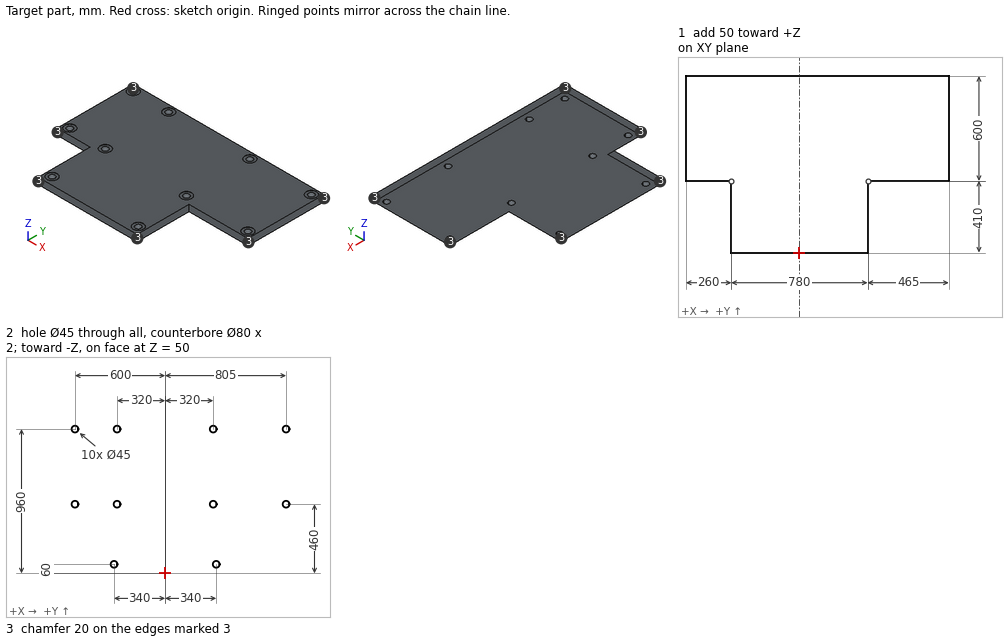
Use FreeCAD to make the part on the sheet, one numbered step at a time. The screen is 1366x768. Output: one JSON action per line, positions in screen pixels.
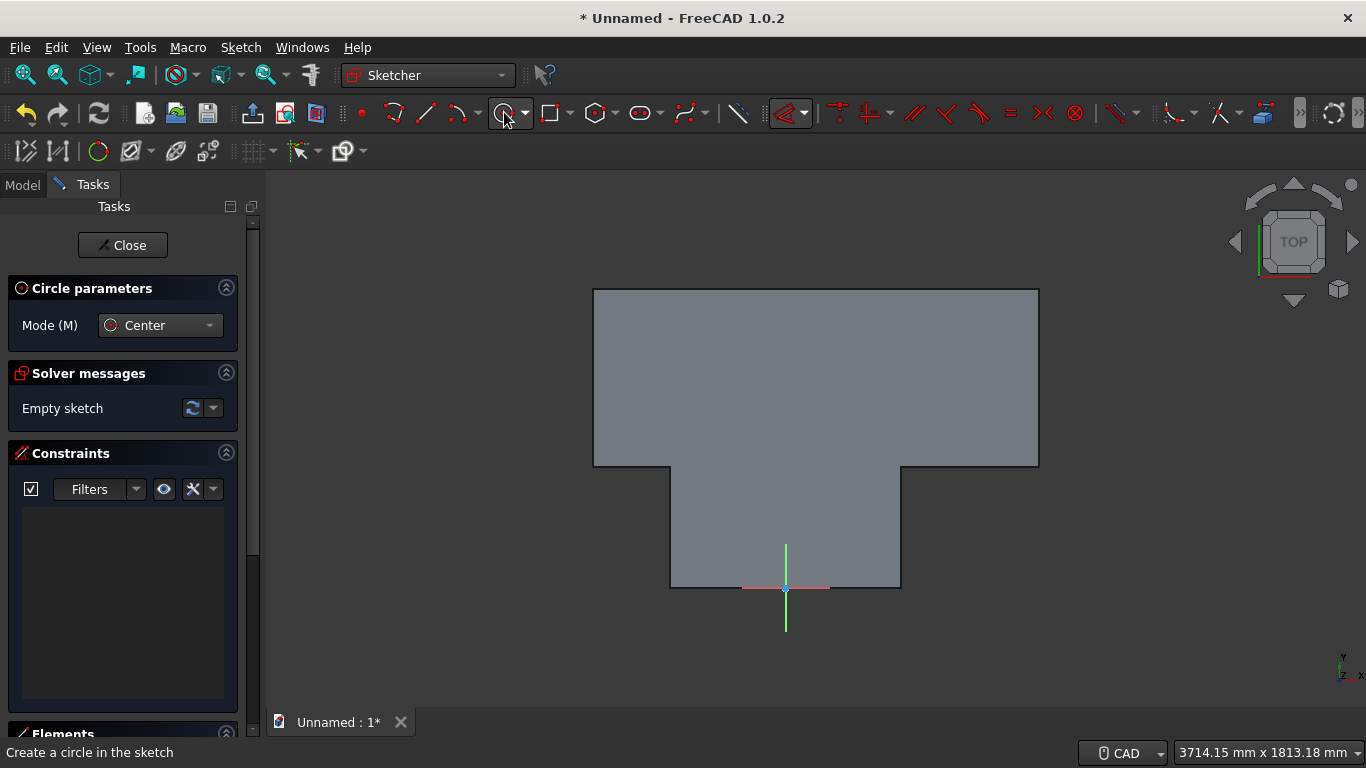
{"action": "scroll", "coordinate": [608, 304], "scroll_direction": "up", "scroll_amount": 7}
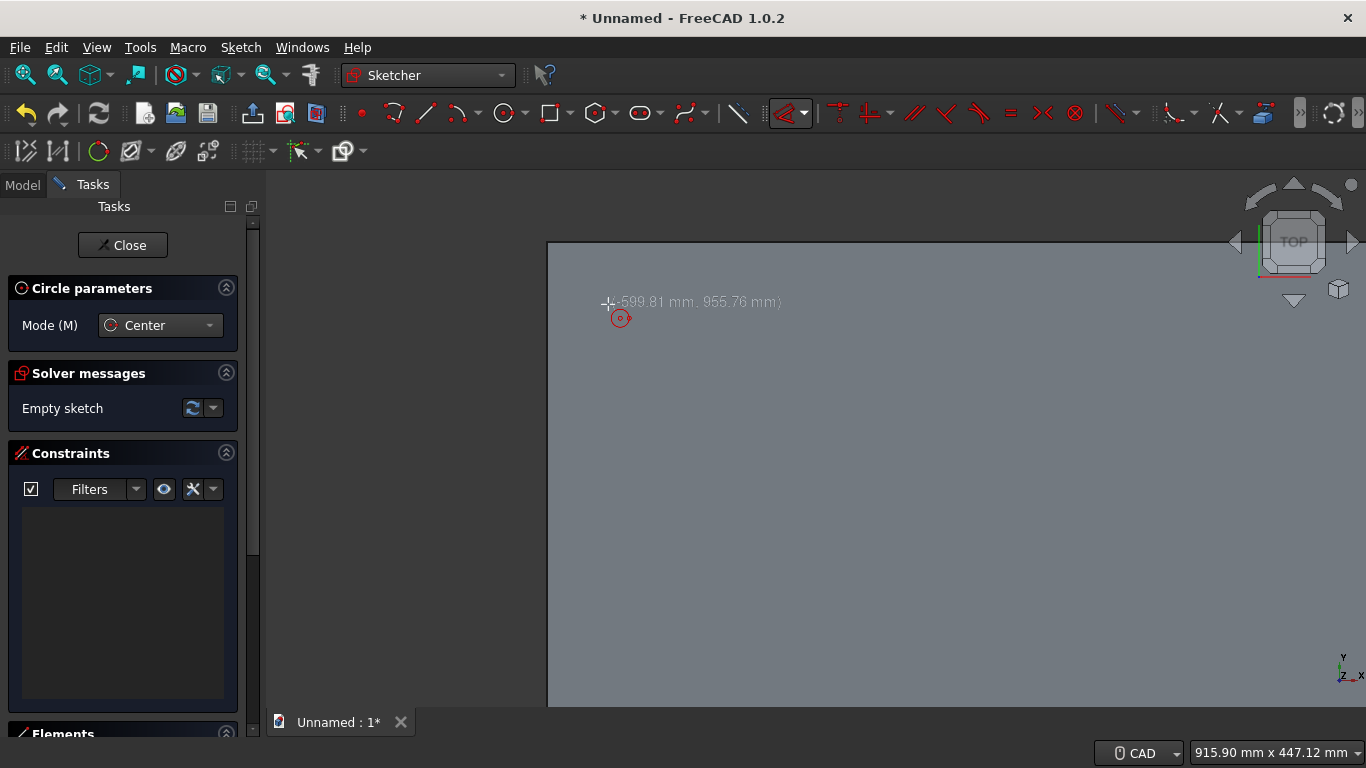
{"action": "scroll", "coordinate": [444, 255], "scroll_direction": "down", "scroll_amount": 6}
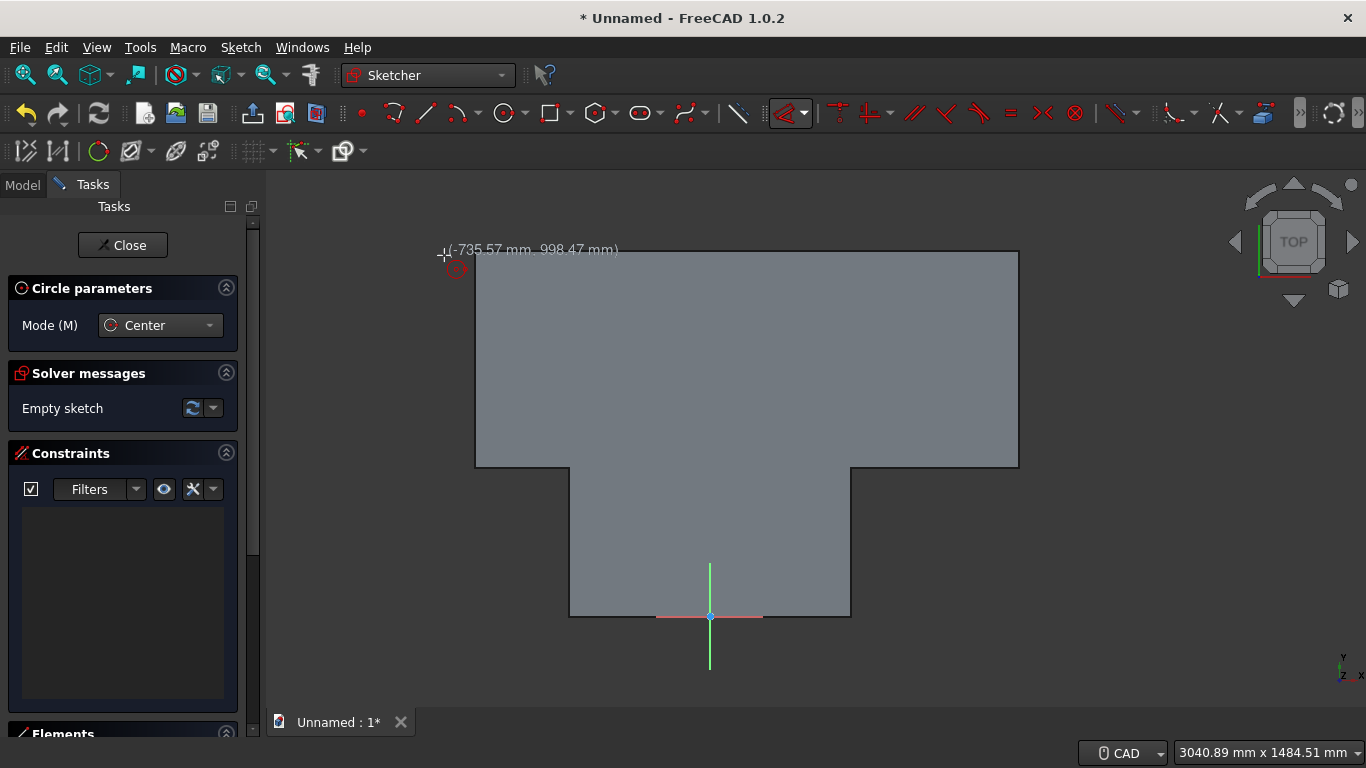
{"action": "left_click", "coordinate": [493, 269]}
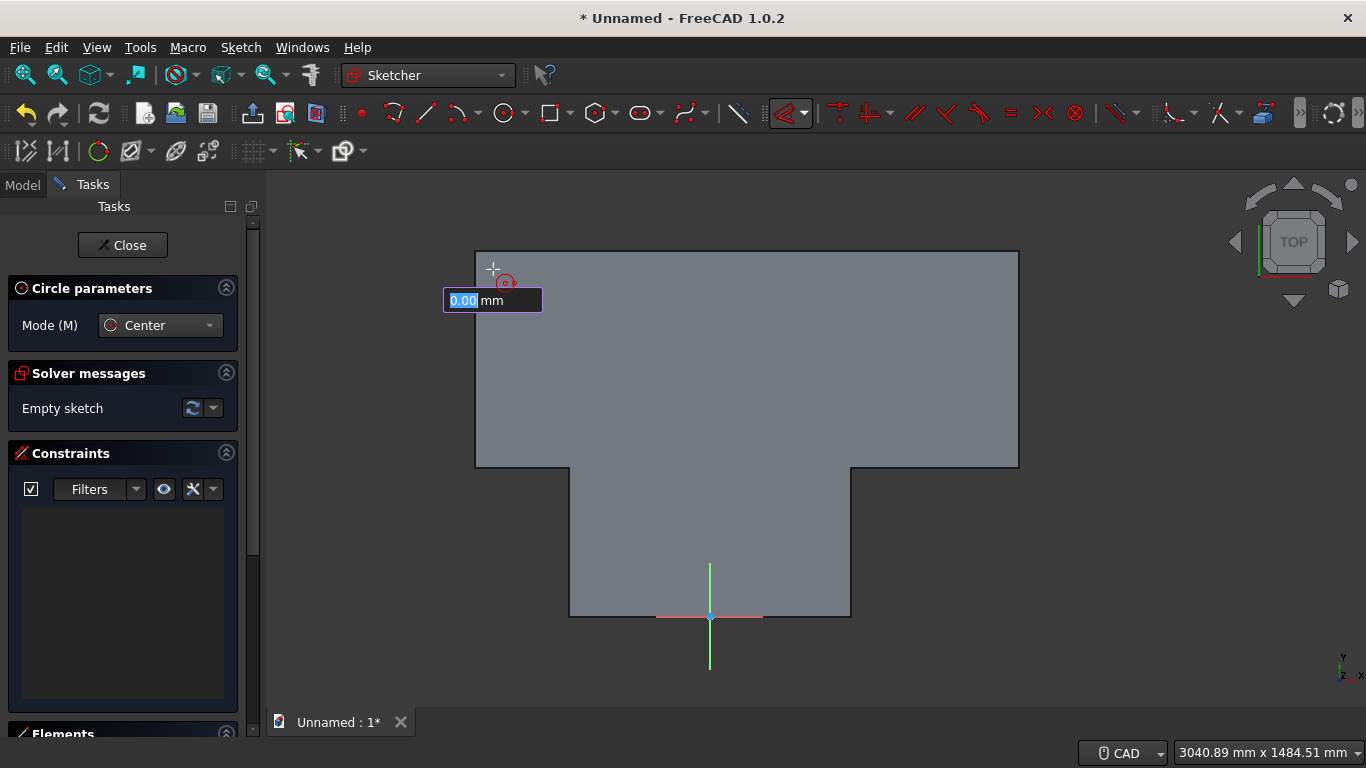
{"action": "scroll", "coordinate": [499, 264], "scroll_direction": "up", "scroll_amount": 4}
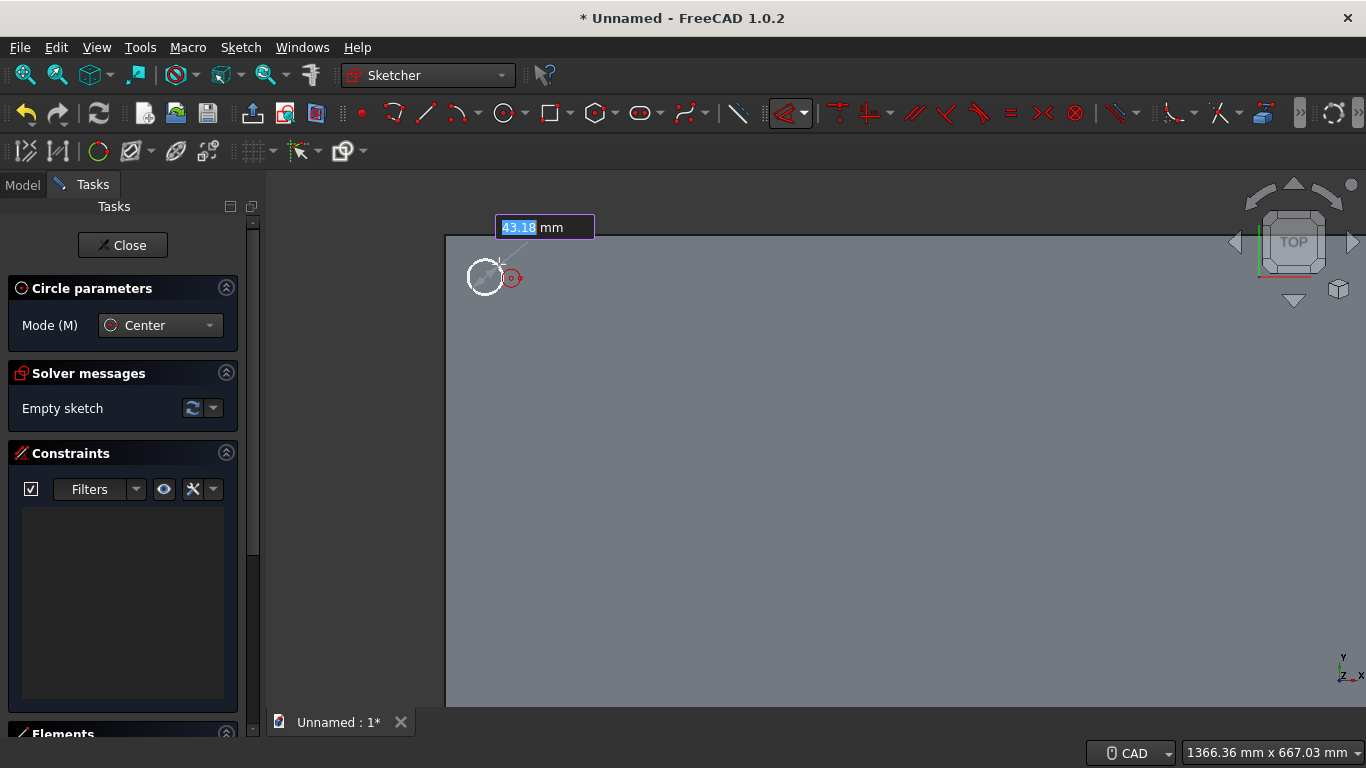
{"action": "left_click", "coordinate": [499, 263]}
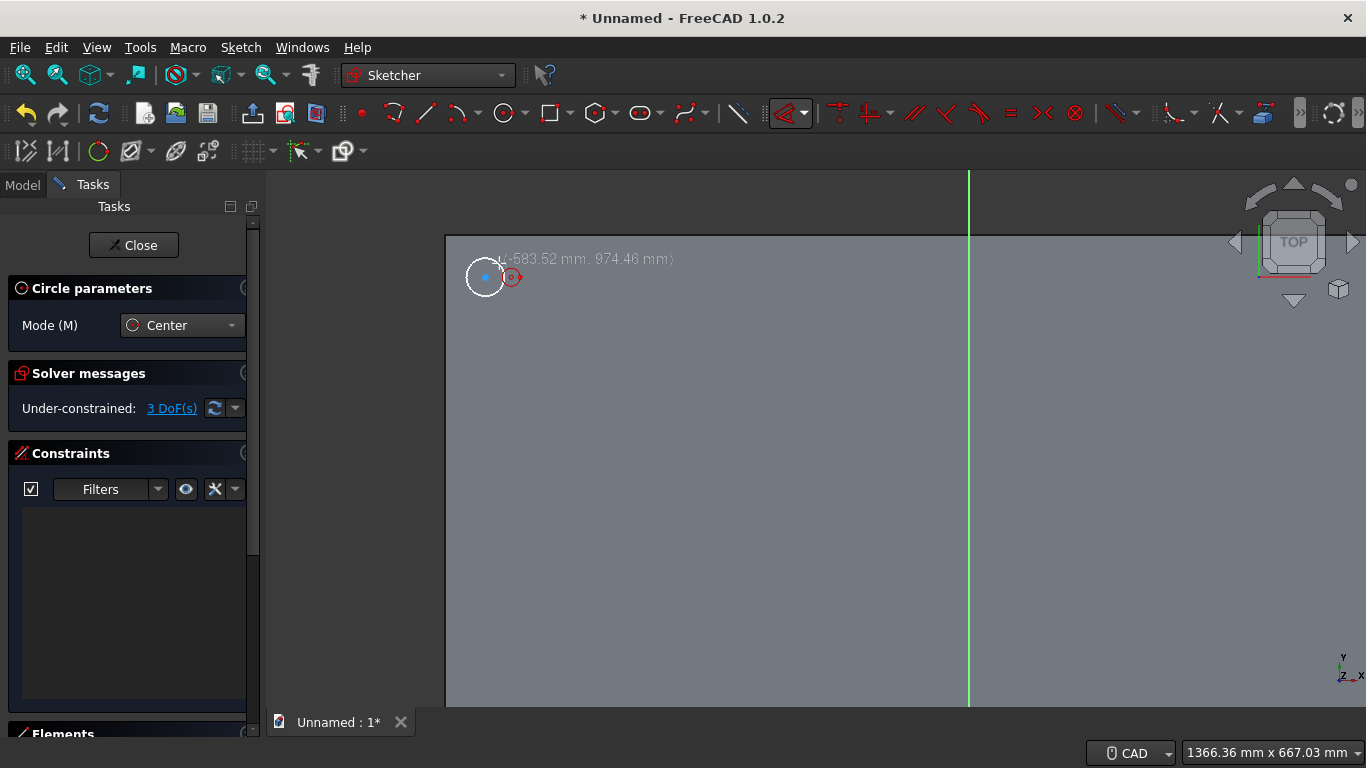
{"action": "scroll", "coordinate": [500, 263], "scroll_direction": "down", "scroll_amount": 4}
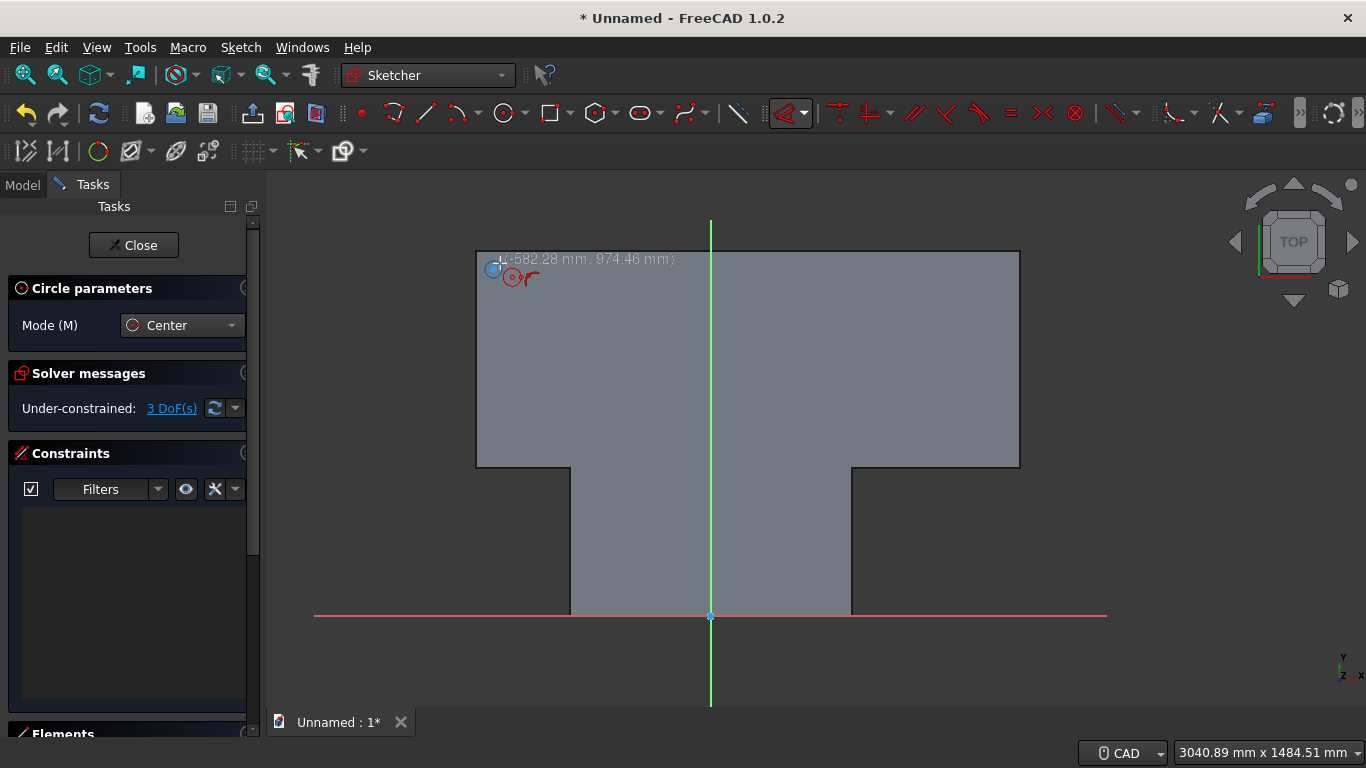
{"action": "scroll", "coordinate": [827, 269], "scroll_direction": "up", "scroll_amount": 6}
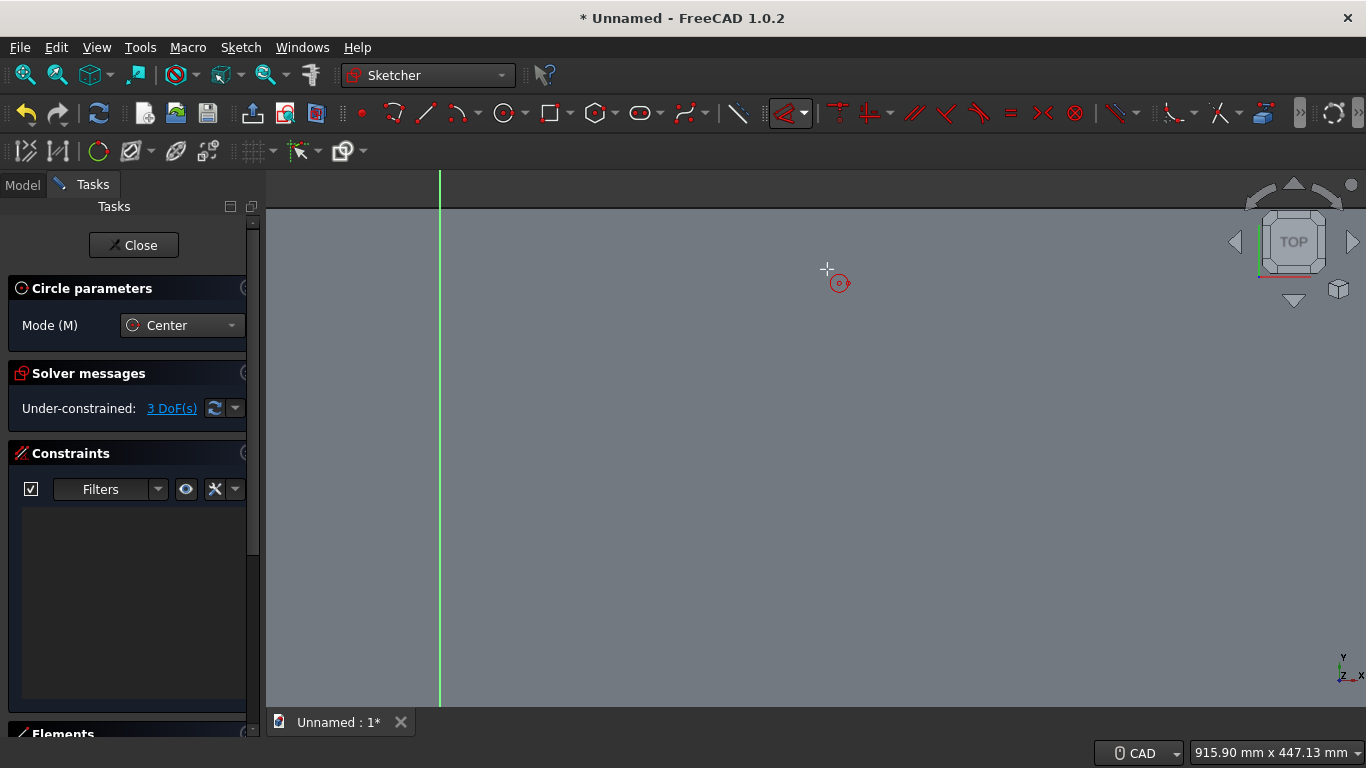
{"action": "scroll", "coordinate": [827, 269], "scroll_direction": "down", "scroll_amount": 6}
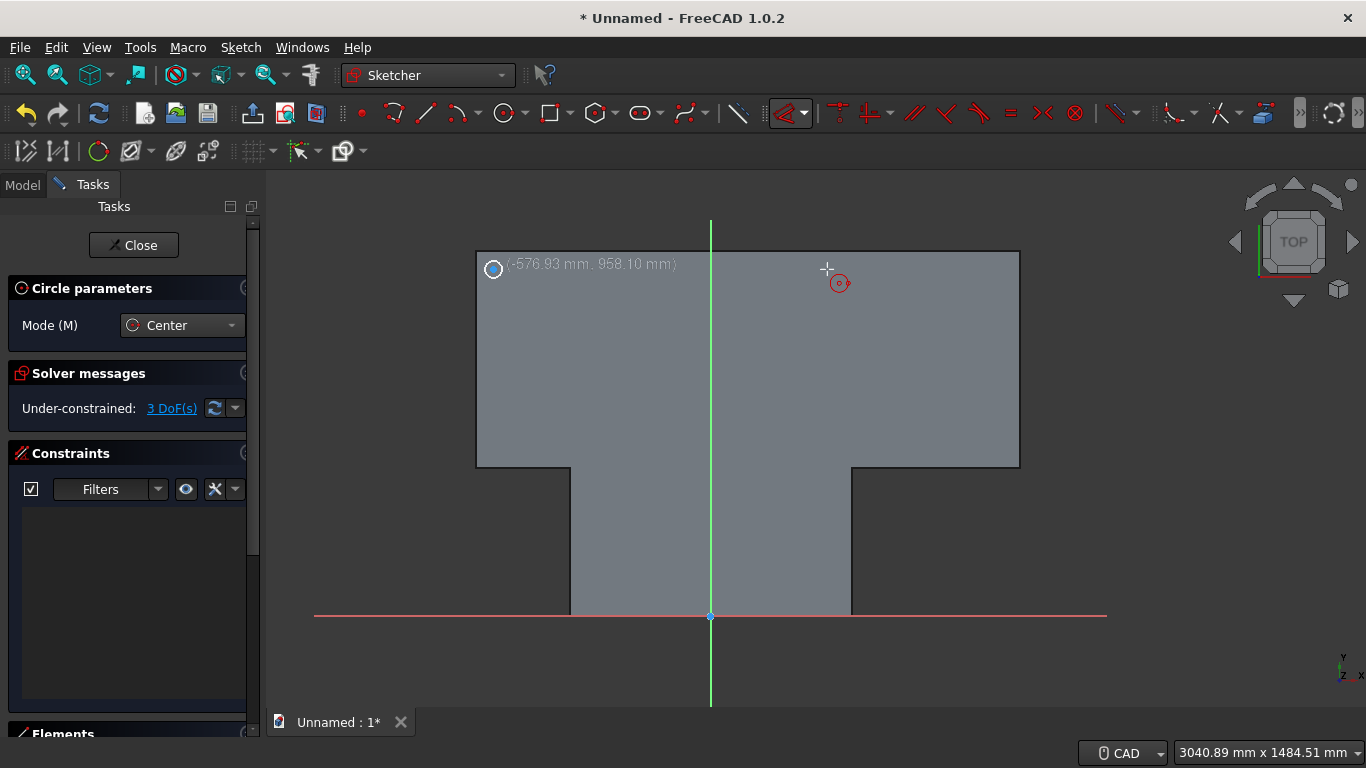
{"action": "left_click", "coordinate": [827, 269]}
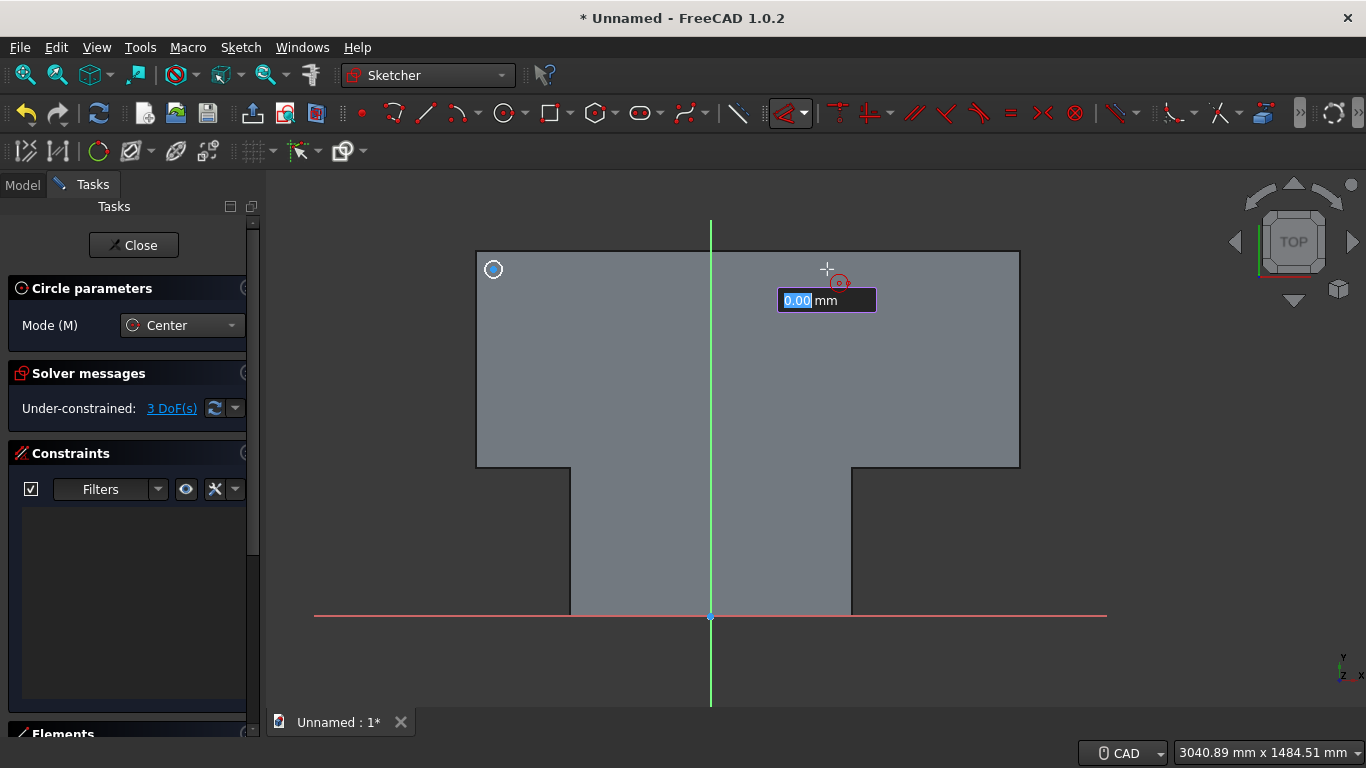
{"action": "scroll", "coordinate": [832, 263], "scroll_direction": "up", "scroll_amount": 4}